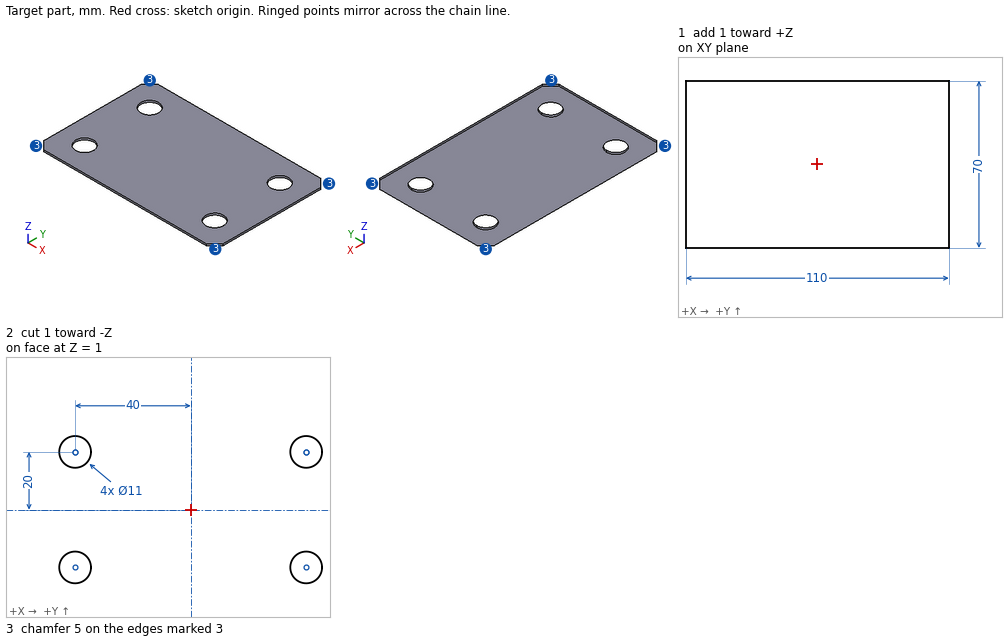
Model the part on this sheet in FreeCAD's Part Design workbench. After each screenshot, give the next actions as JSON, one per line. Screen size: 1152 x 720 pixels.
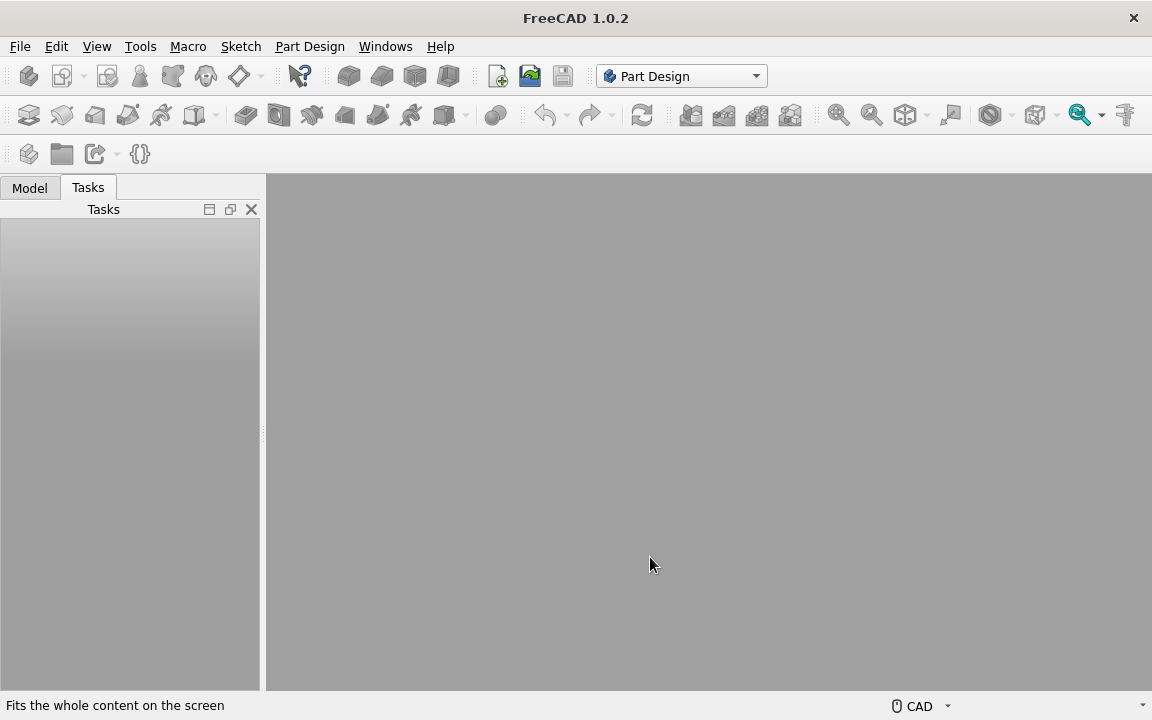
{"action": "left_click", "coordinate": [497, 76]}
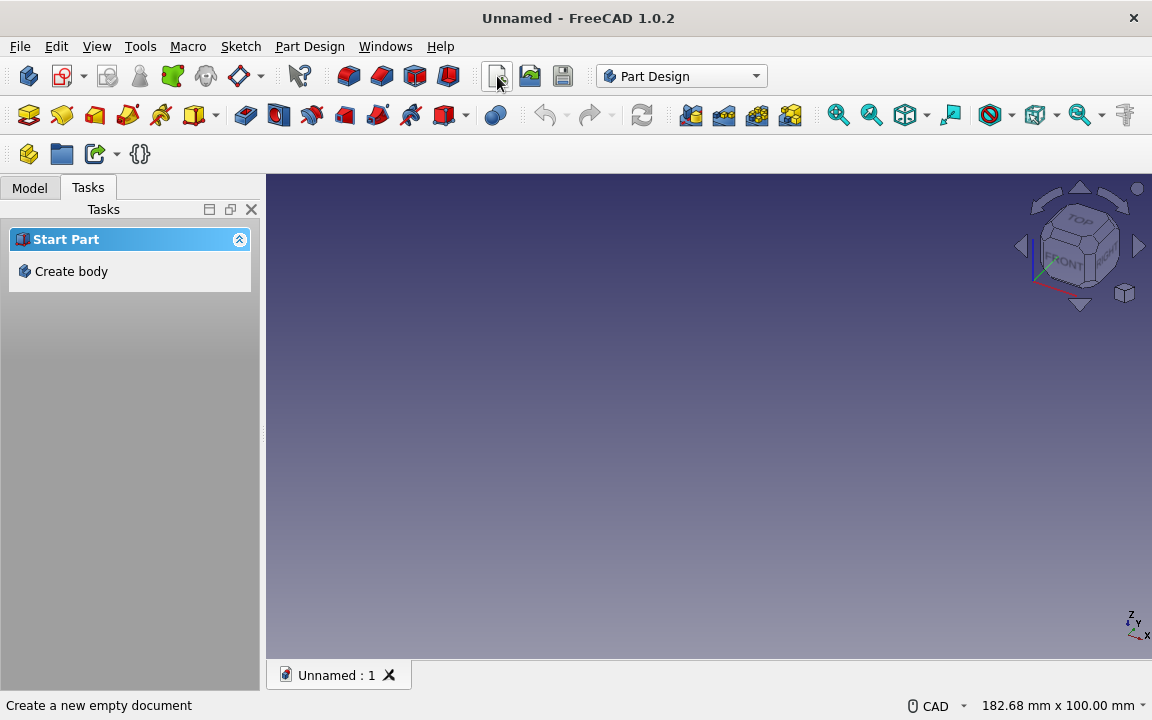
{"action": "left_click", "coordinate": [62, 76]}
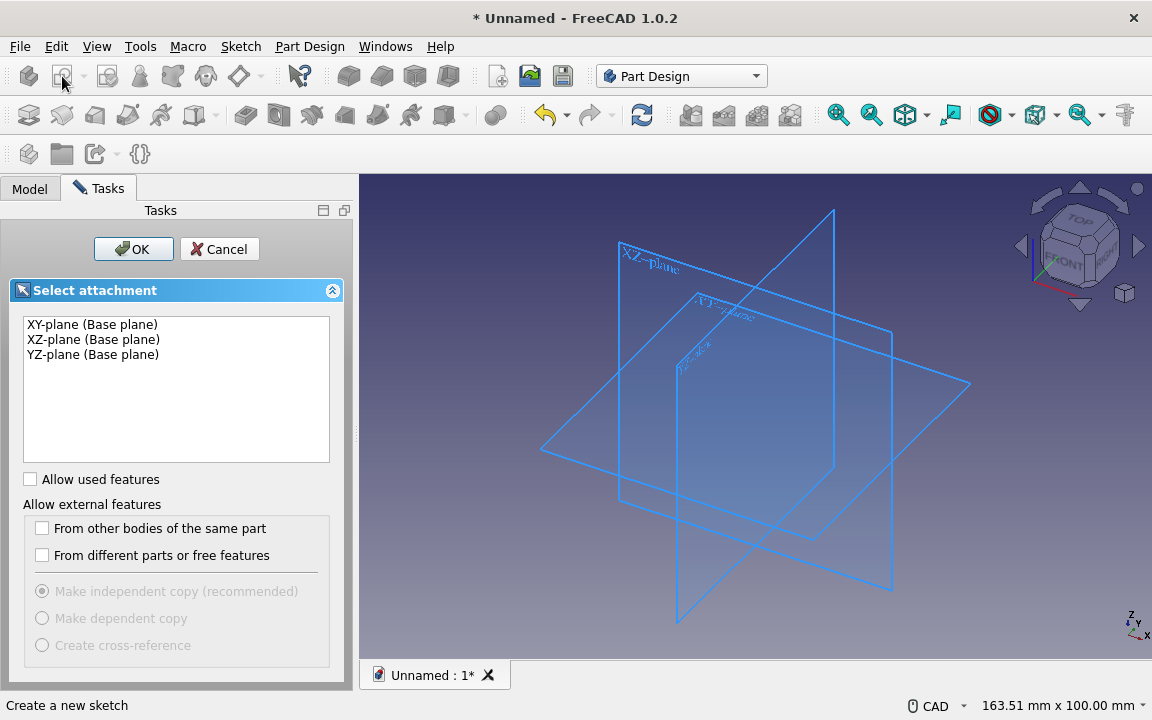
{"action": "left_click", "coordinate": [84, 324]}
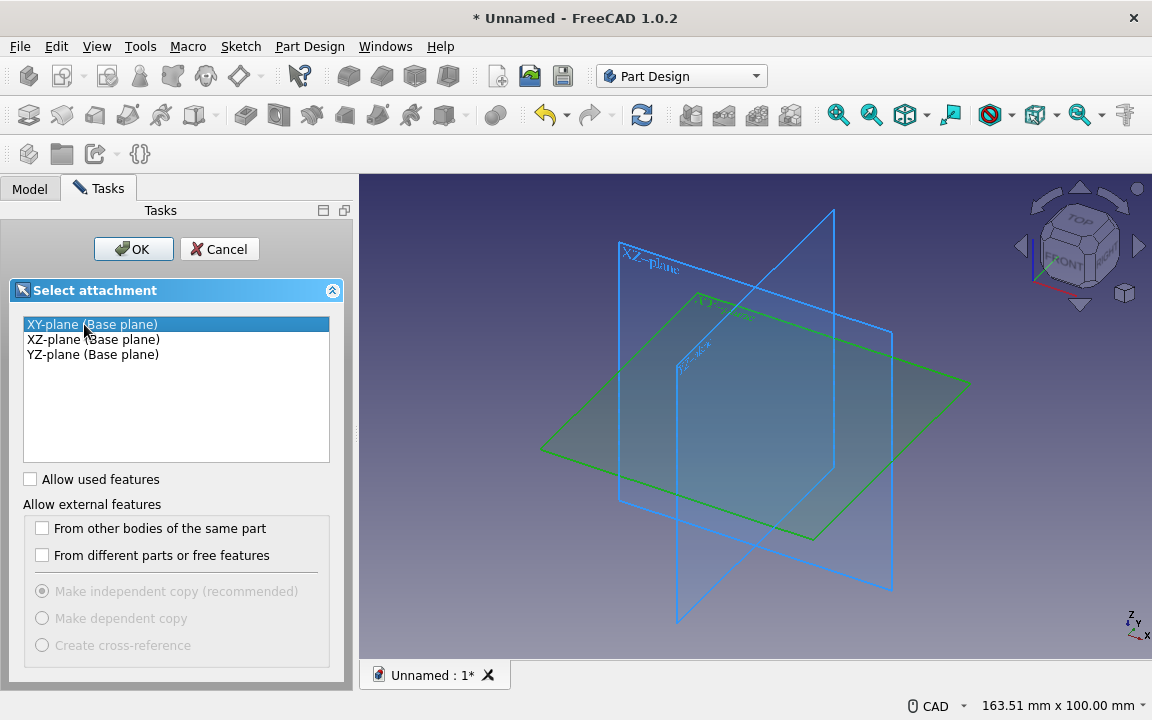
{"action": "left_click", "coordinate": [134, 249]}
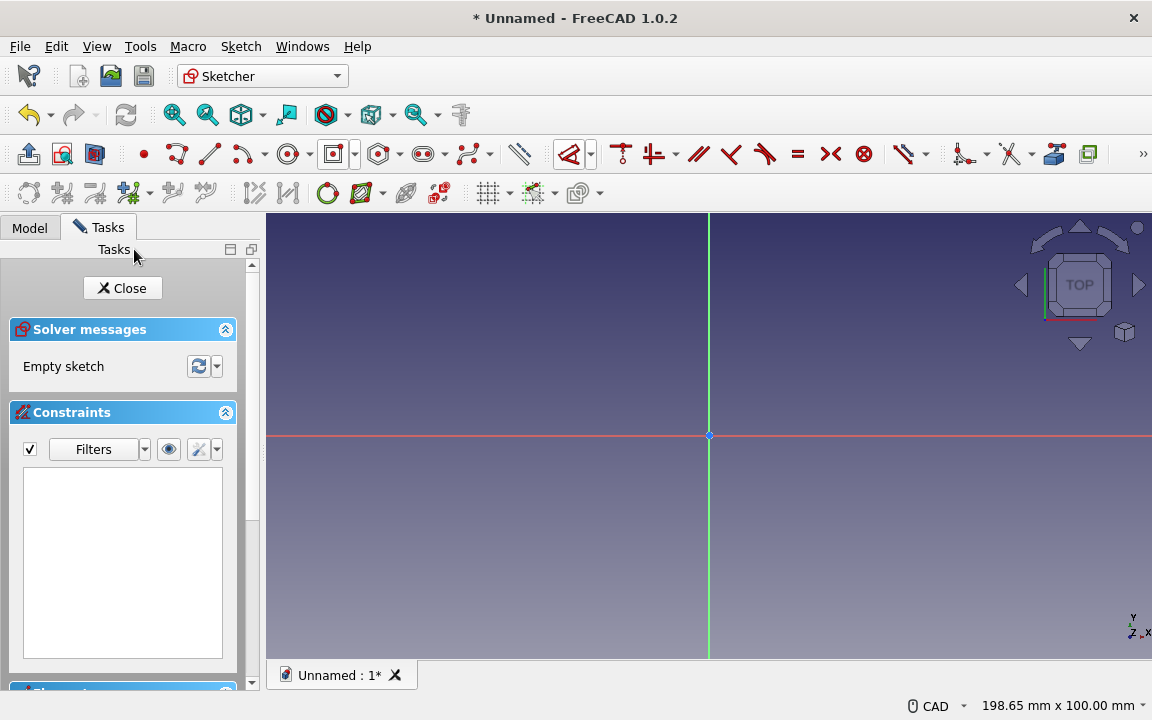
{"action": "left_click", "coordinate": [332, 154]}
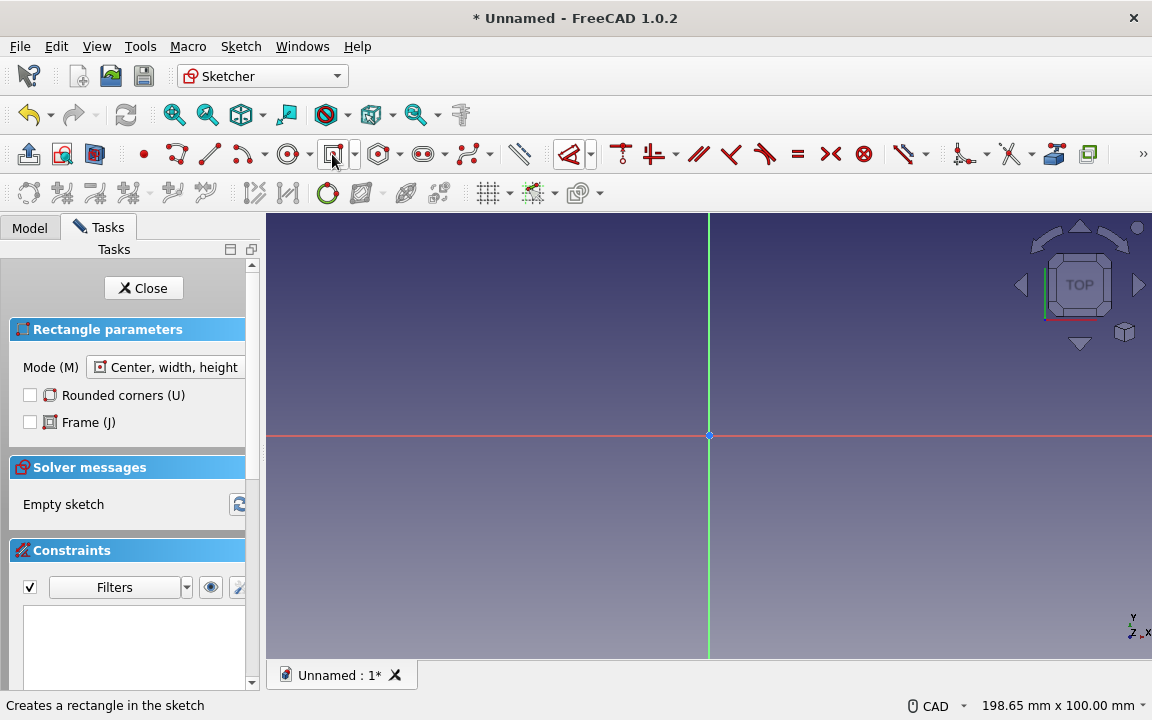
{"action": "left_click", "coordinate": [709, 436]}
{"action": "mouse_move", "coordinate": [954, 280]}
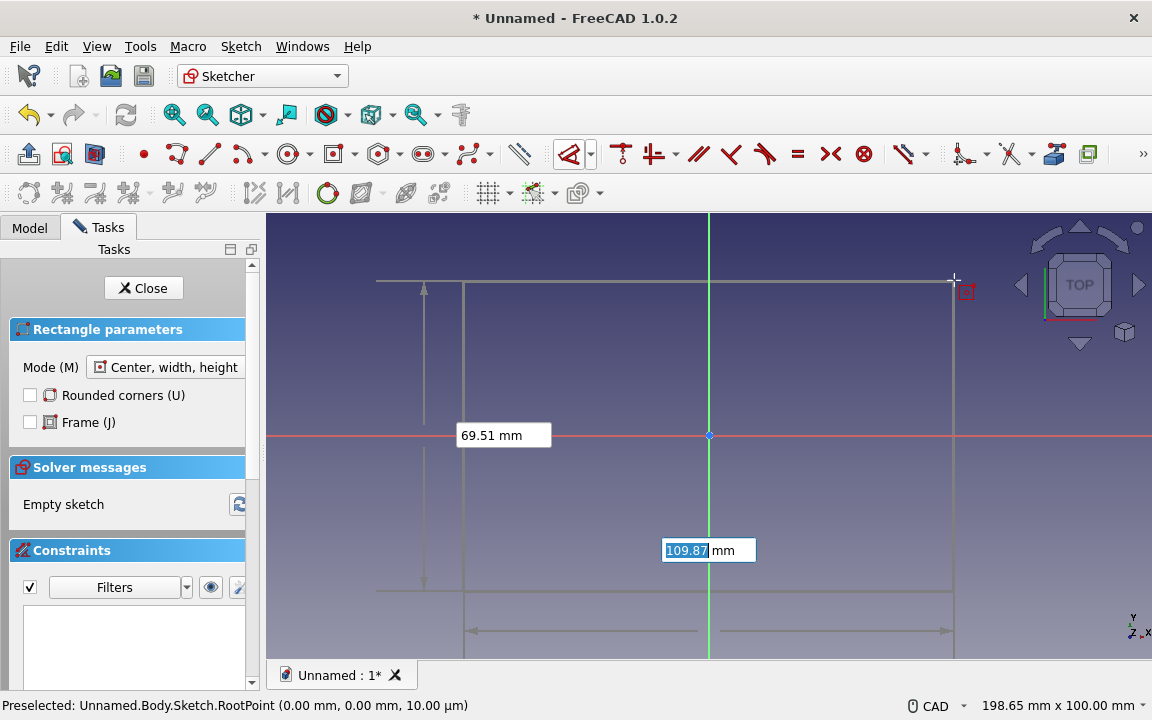
{"action": "type", "text": "110"}
{"action": "key", "text": "Tab"}
{"action": "type", "text": "70"}
{"action": "key", "text": "Return"}
{"action": "key", "text": "Escape"}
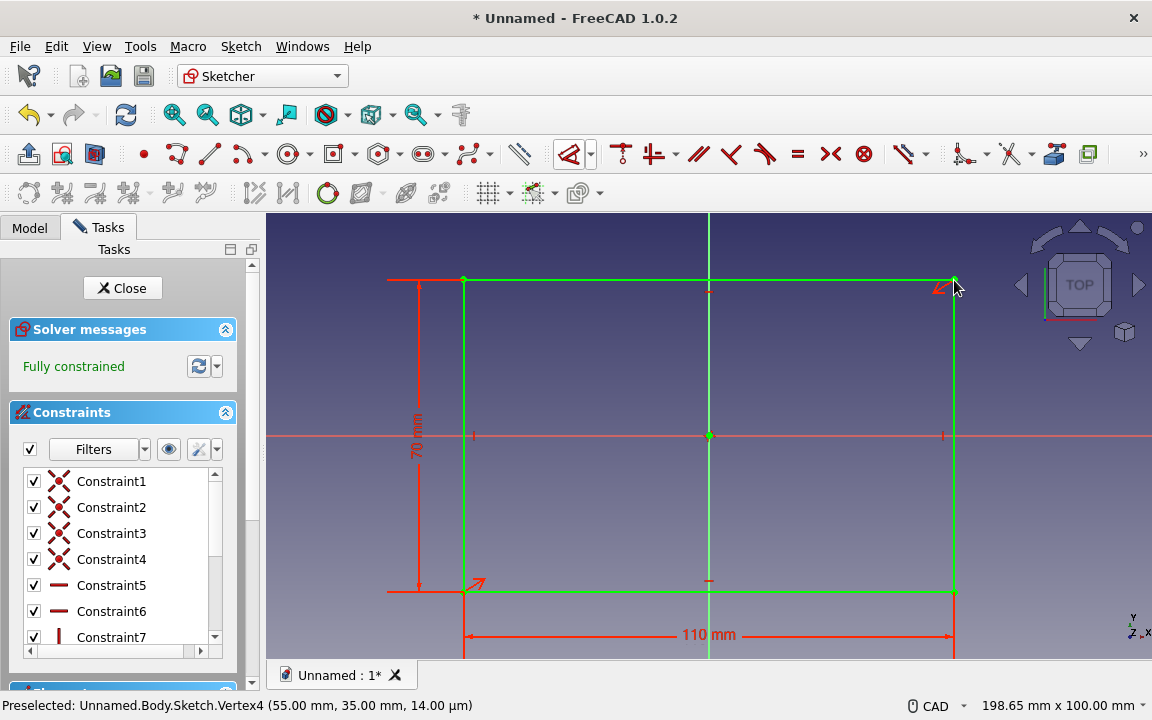
{"action": "left_click", "coordinate": [123, 288]}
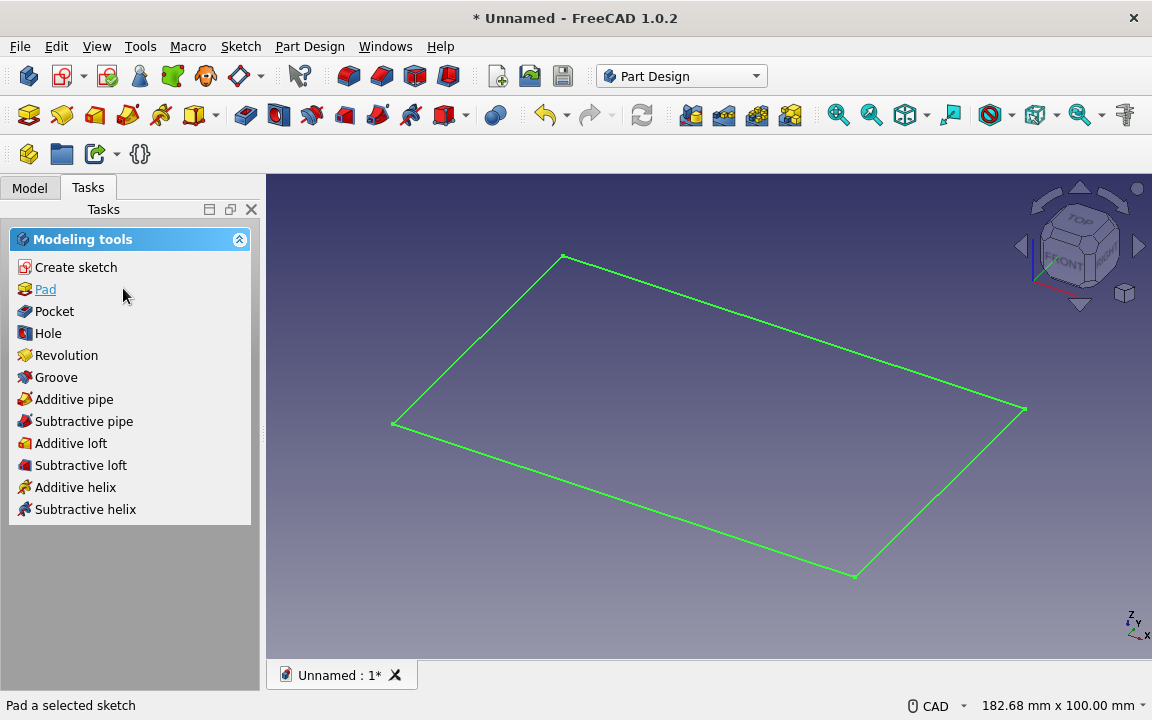
{"action": "left_click", "coordinate": [29, 116]}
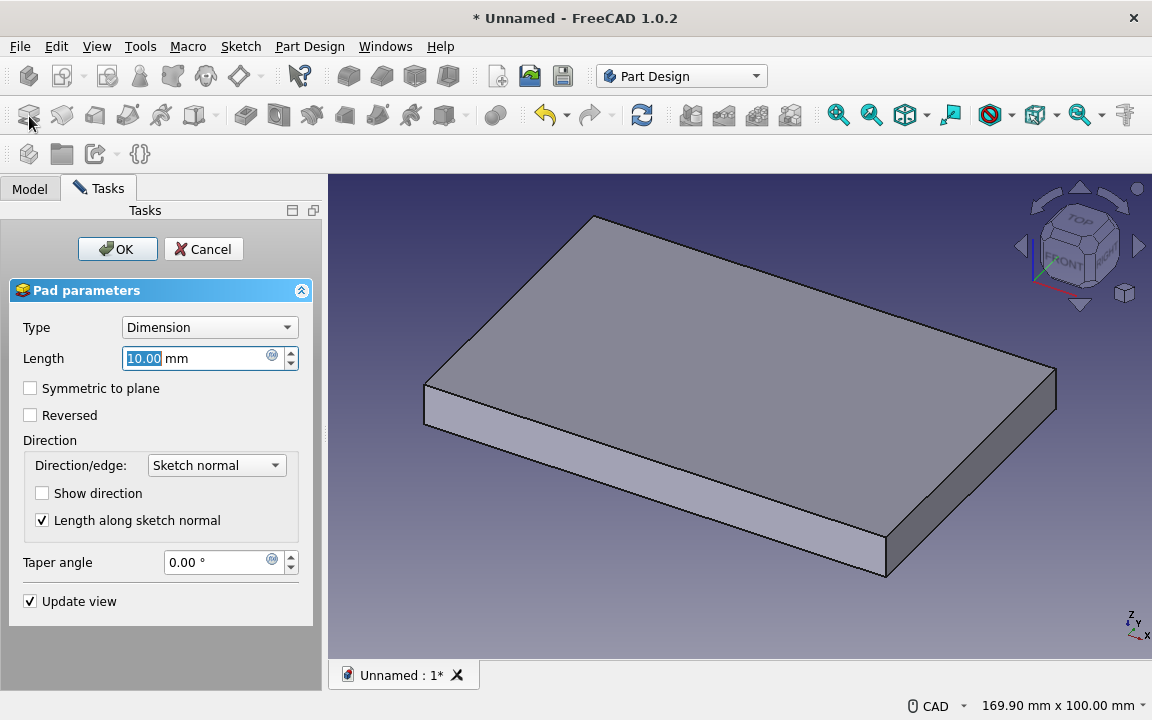
{"action": "type", "text": "1"}
{"action": "key", "text": "Tab"}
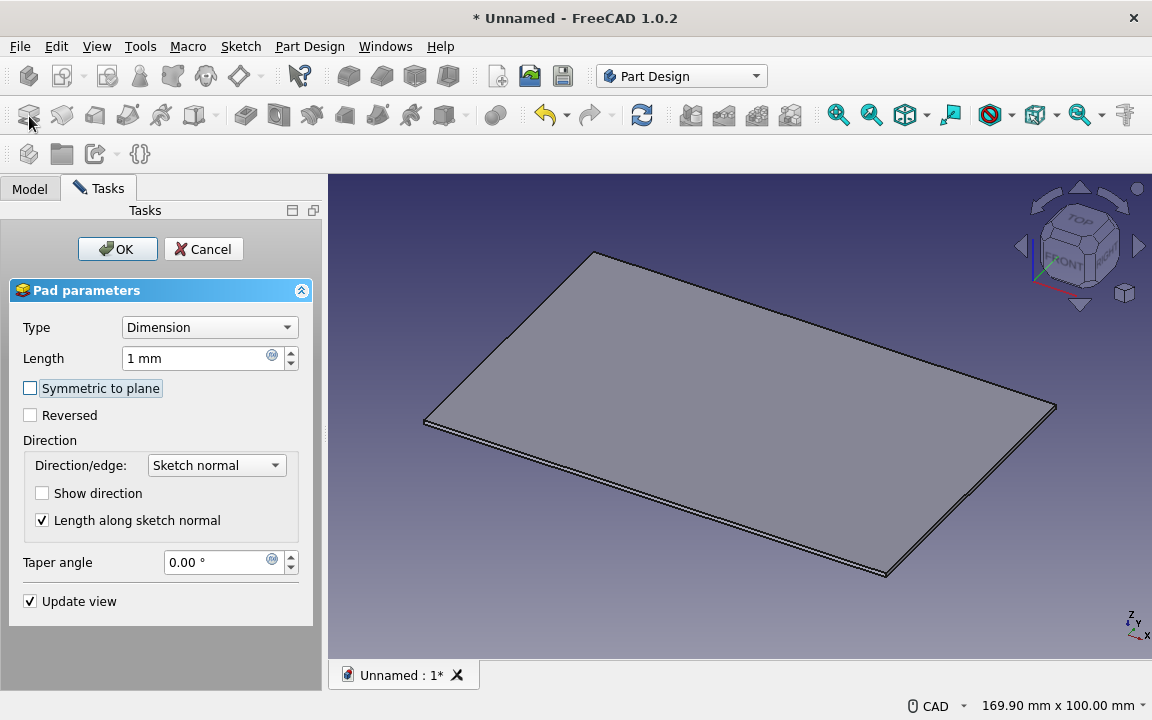
{"action": "left_click", "coordinate": [118, 249]}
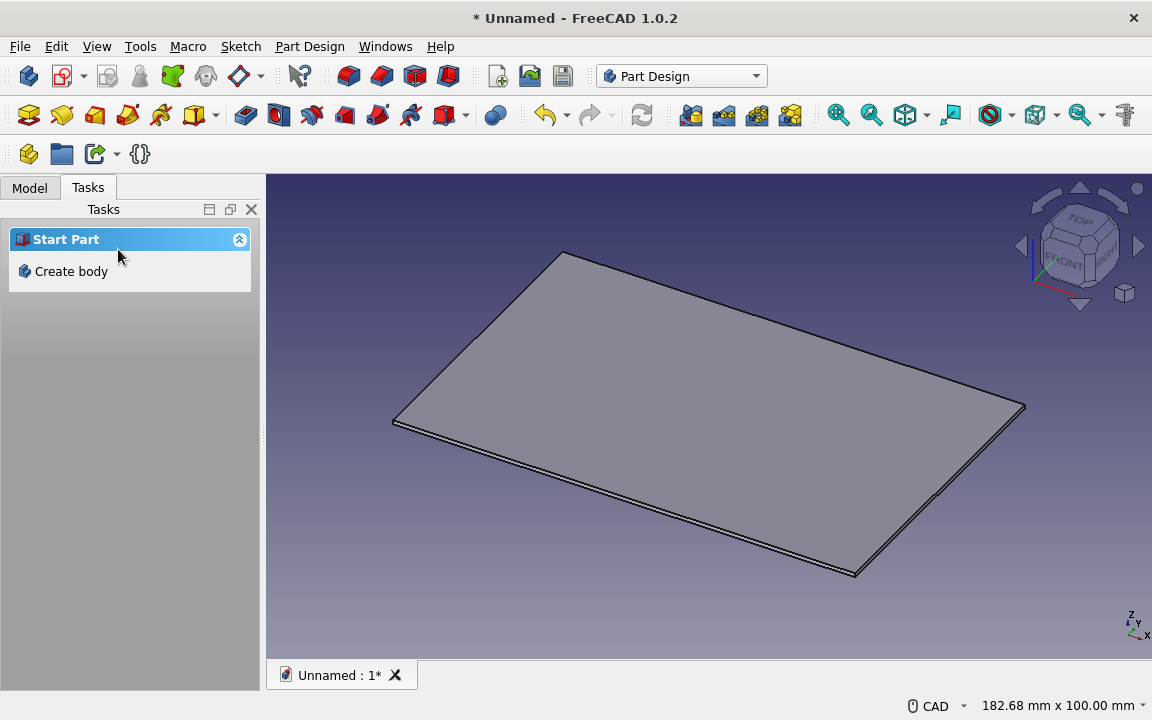
{"action": "left_click", "coordinate": [775, 433]}